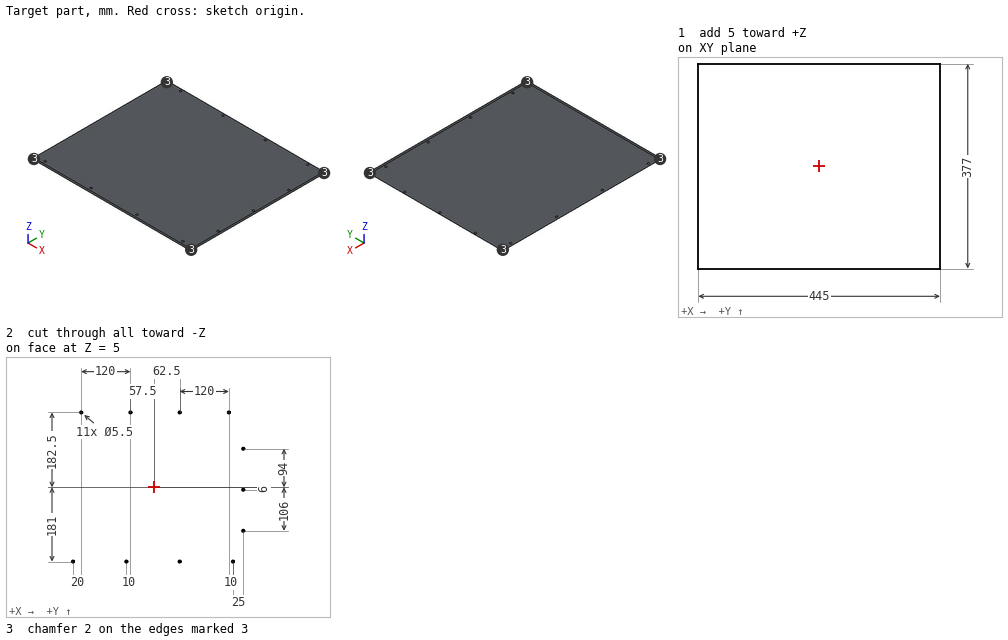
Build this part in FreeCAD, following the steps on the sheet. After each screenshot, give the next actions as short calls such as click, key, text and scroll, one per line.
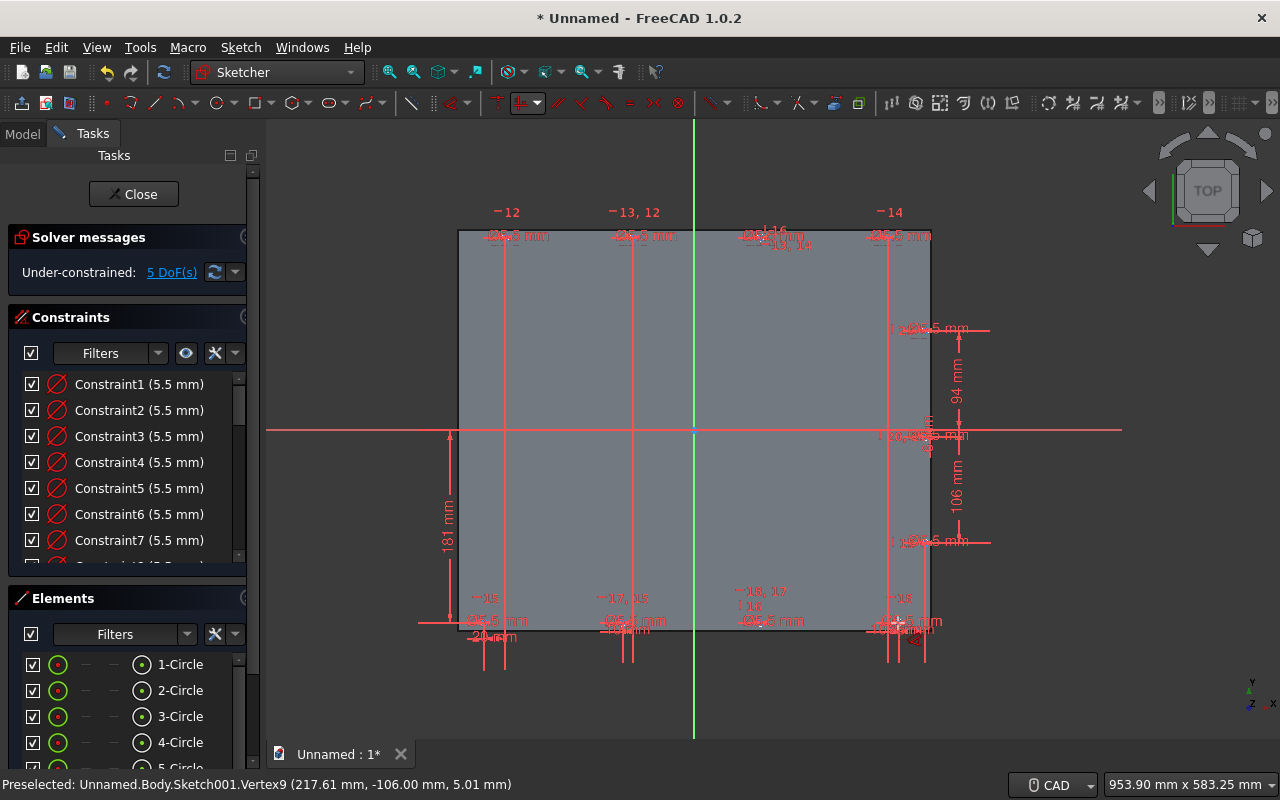
click(633, 238)
click(664, 204)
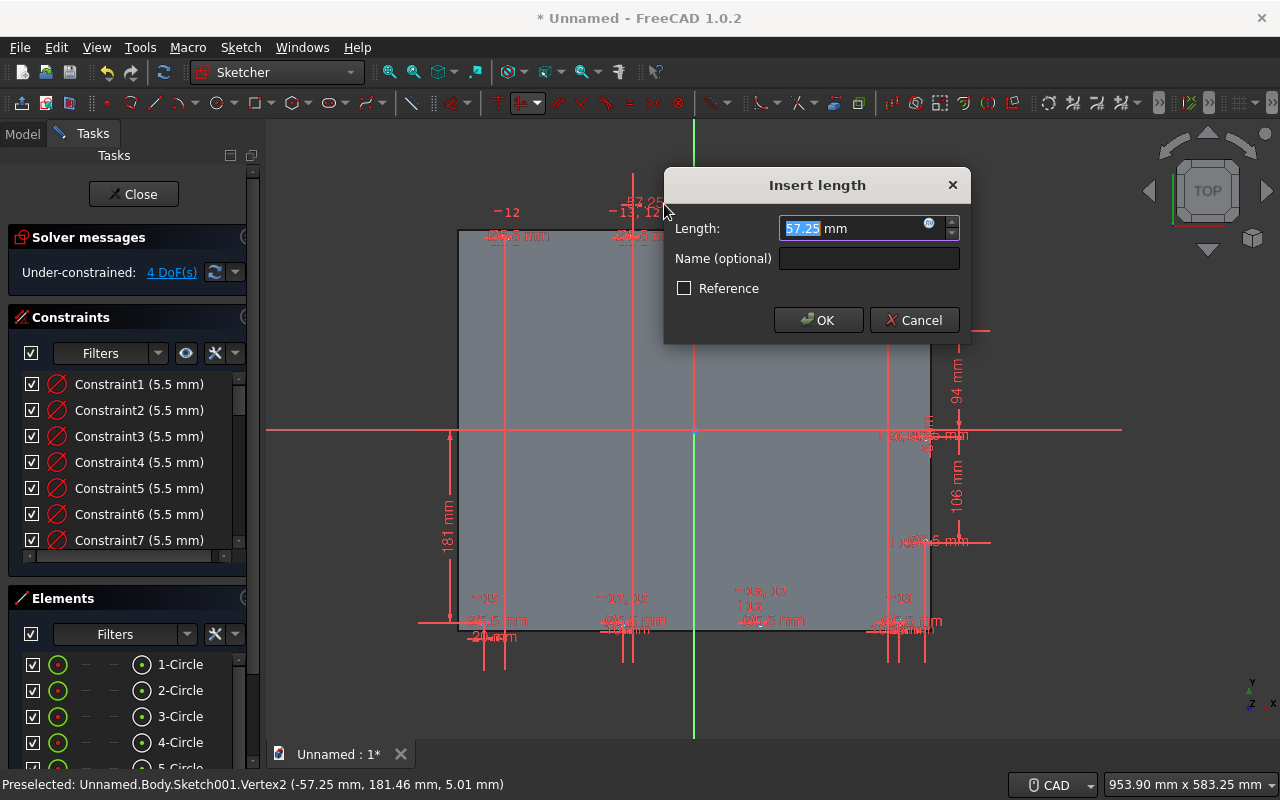
text(57.5)
key(Return)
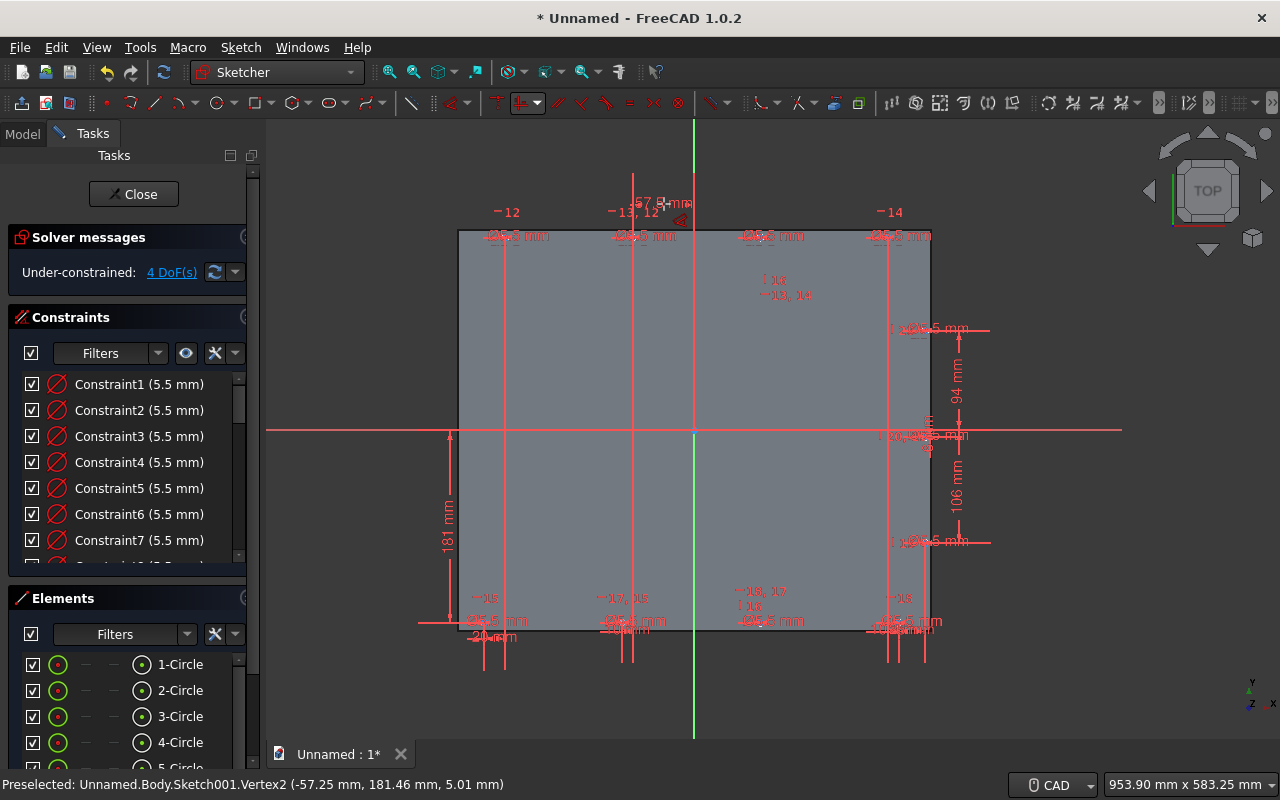
click(760, 238)
click(742, 204)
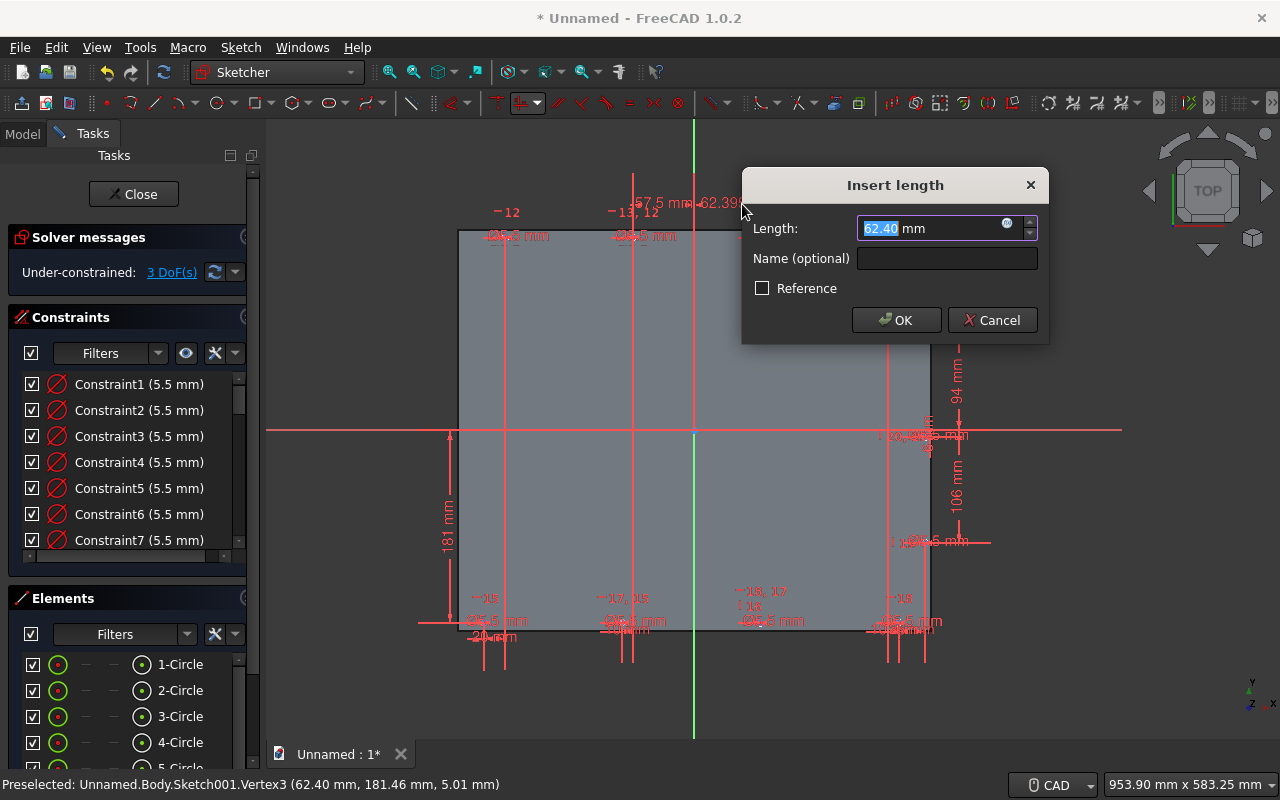
text(62.5)
key(Return)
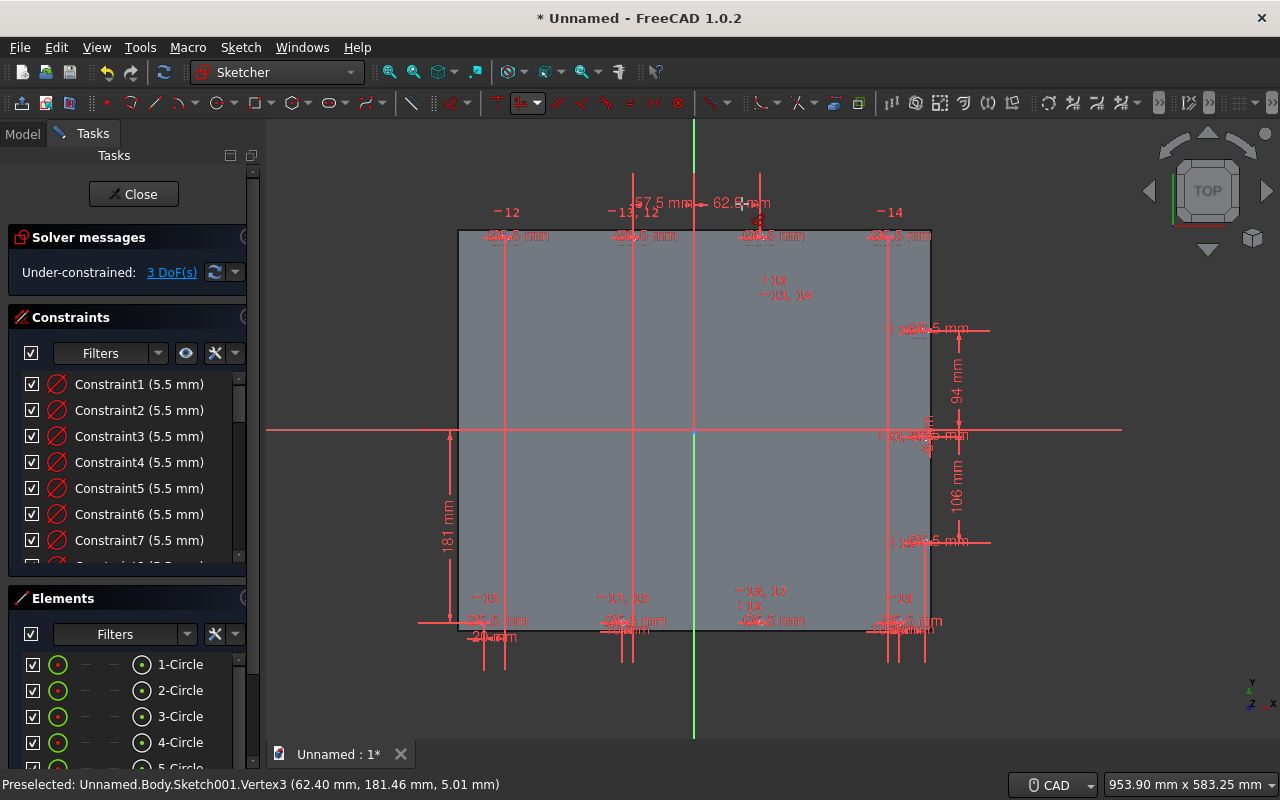
click(505, 238)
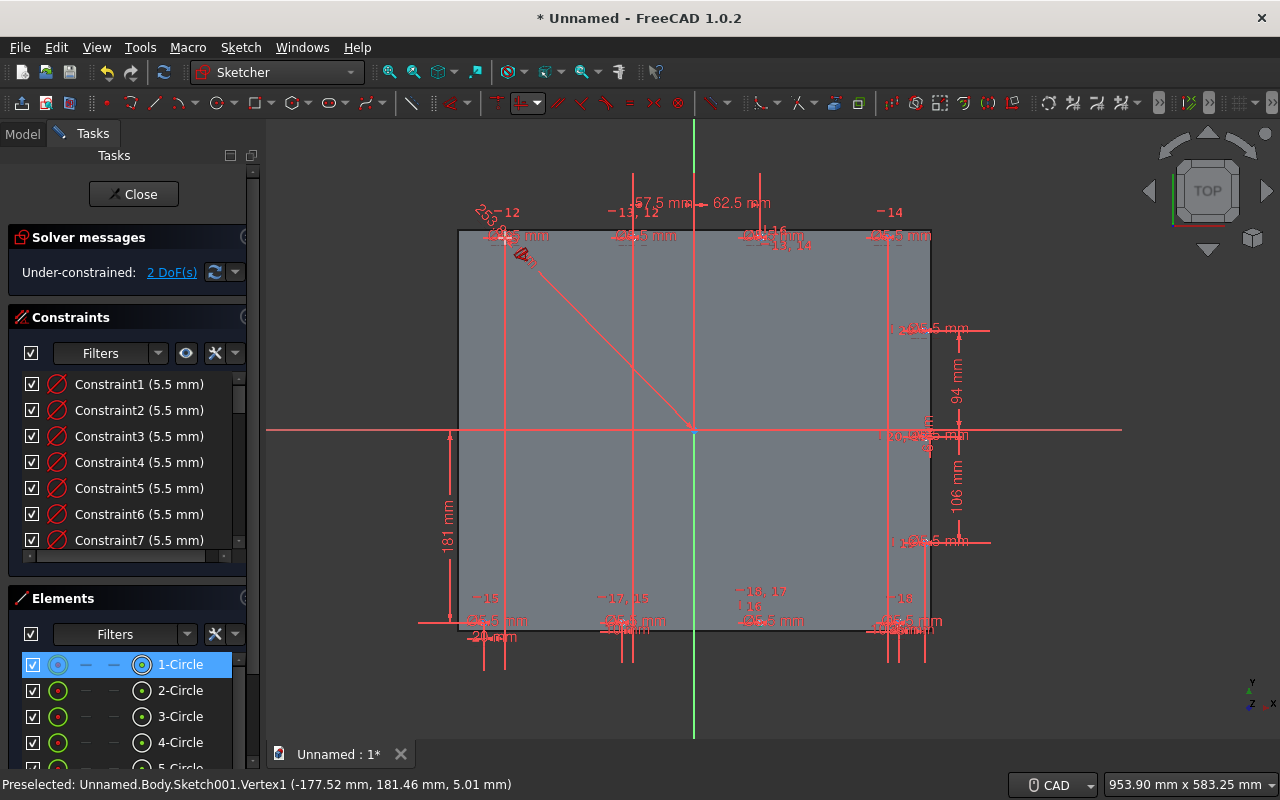
click(633, 238)
click(569, 204)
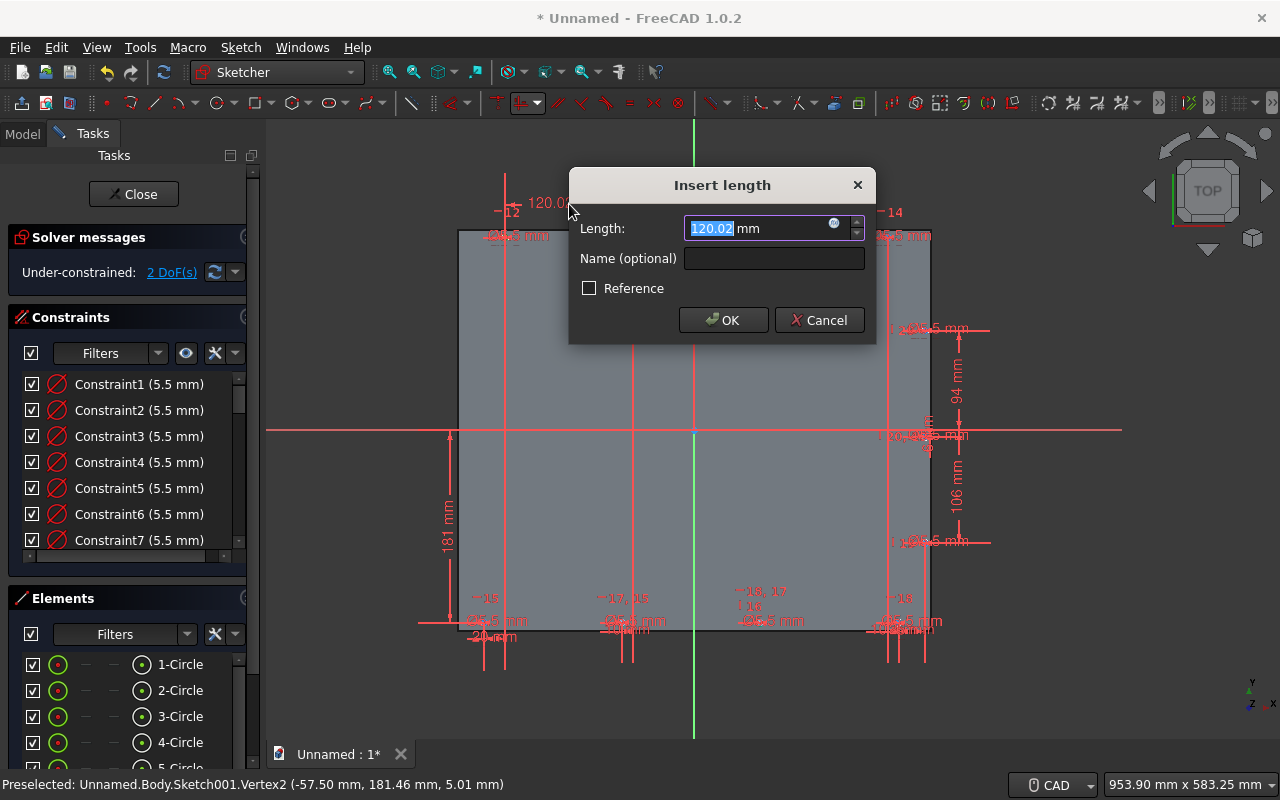
text(120)
key(Return)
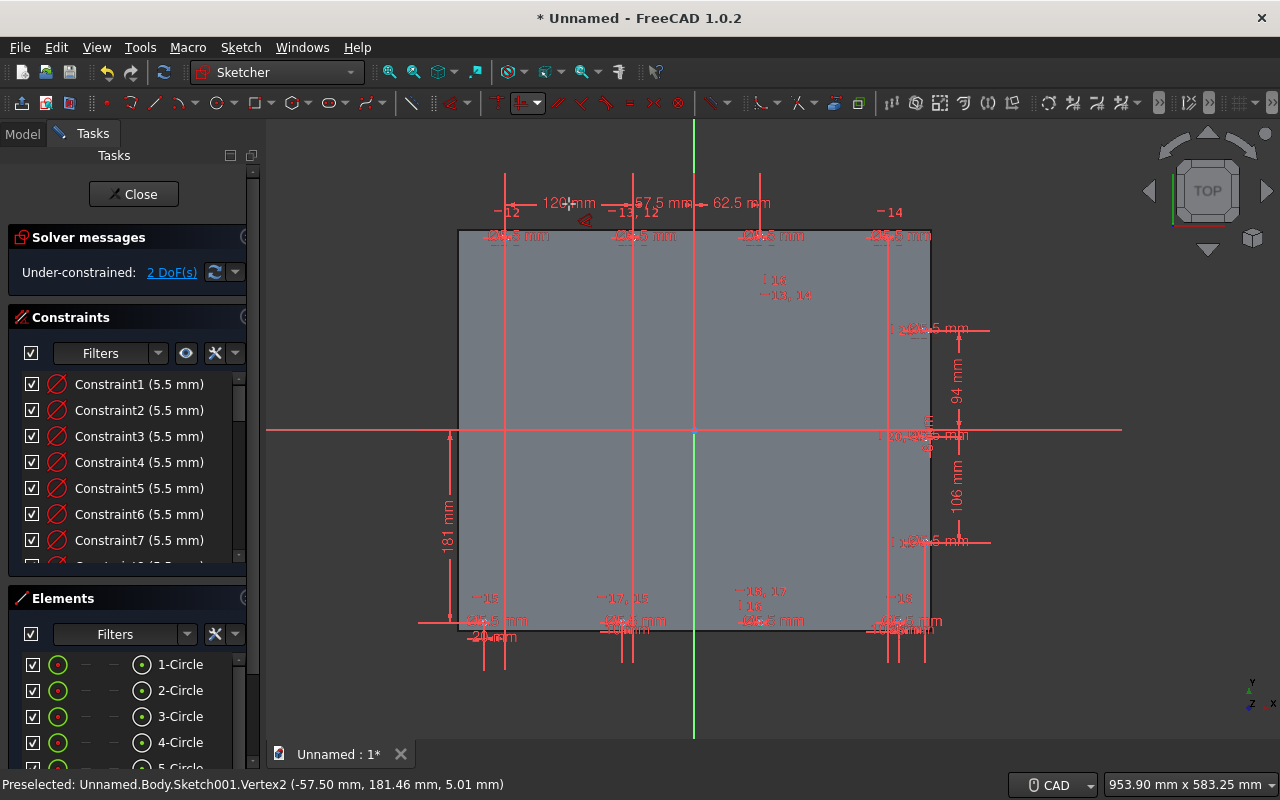
click(760, 238)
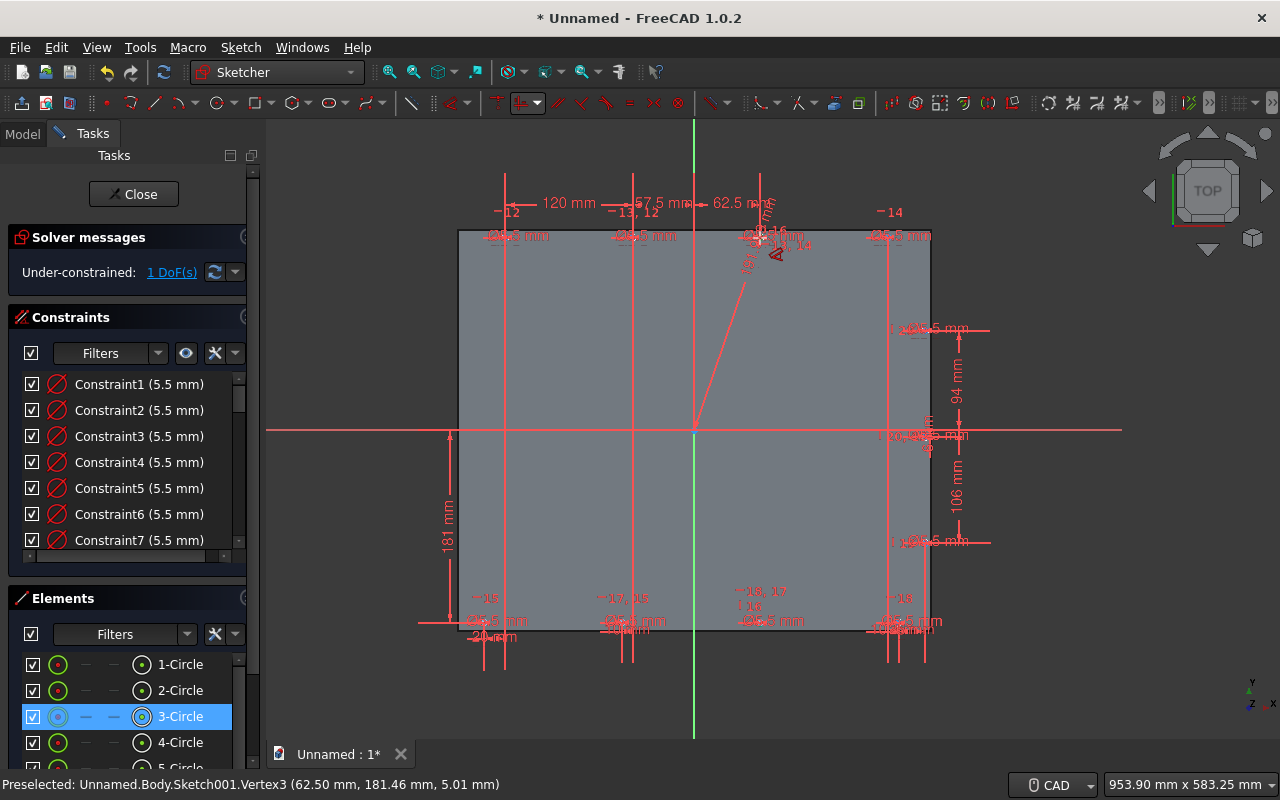
click(888, 238)
click(824, 204)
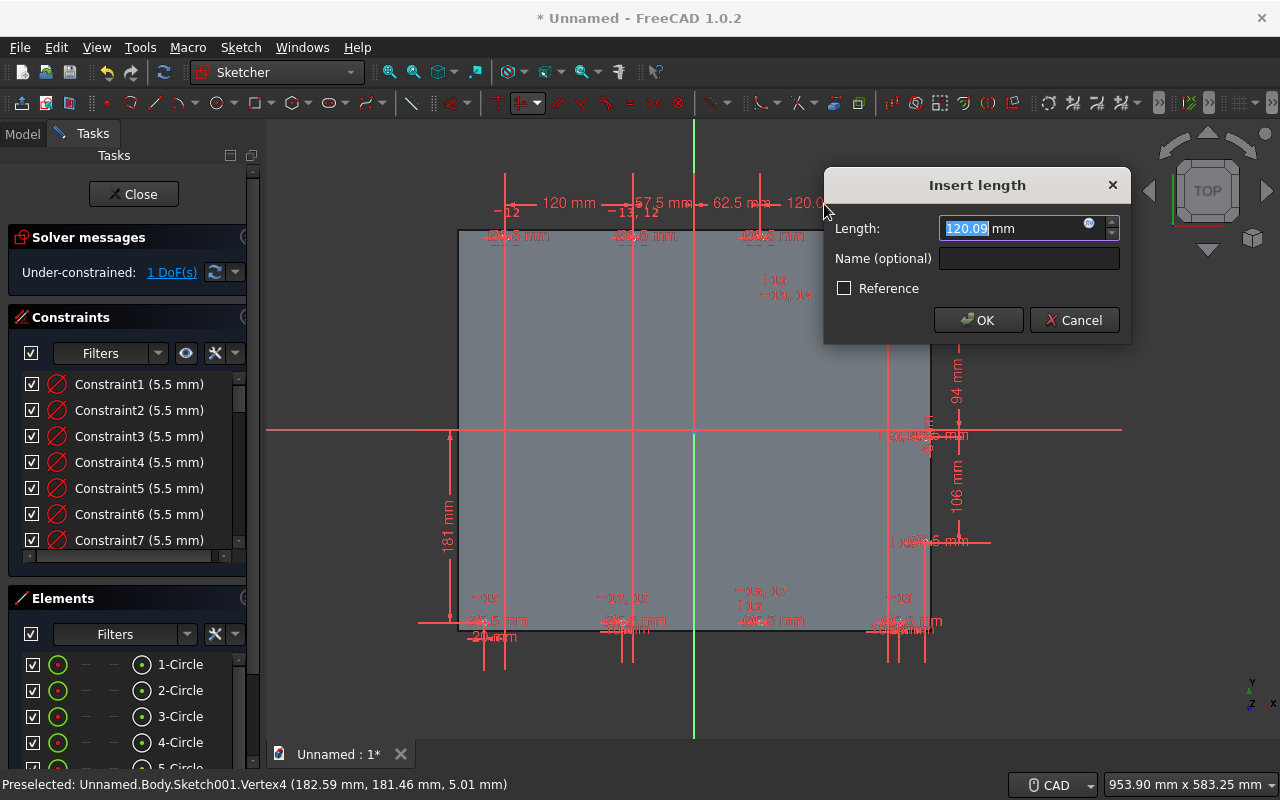
text(120)
key(Return)